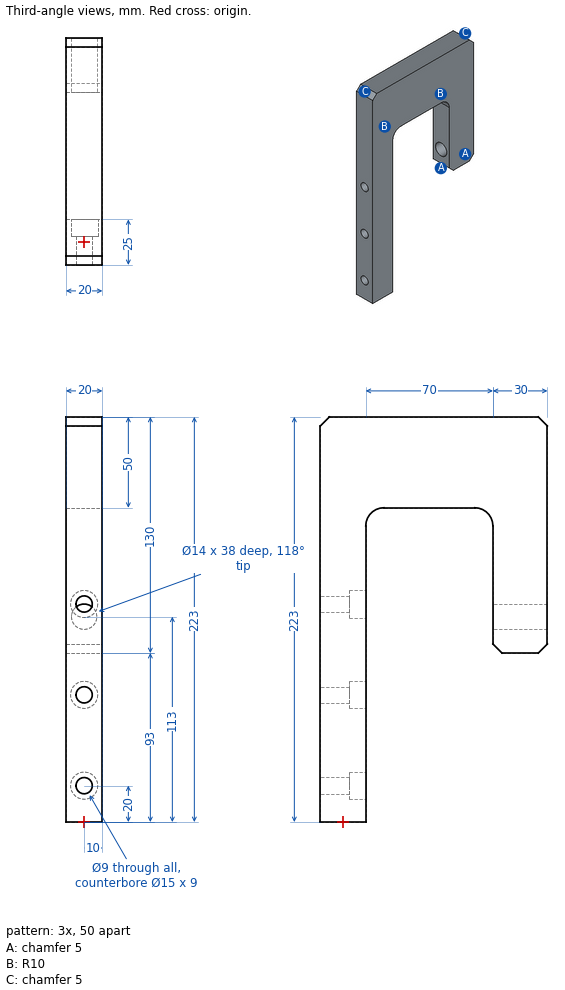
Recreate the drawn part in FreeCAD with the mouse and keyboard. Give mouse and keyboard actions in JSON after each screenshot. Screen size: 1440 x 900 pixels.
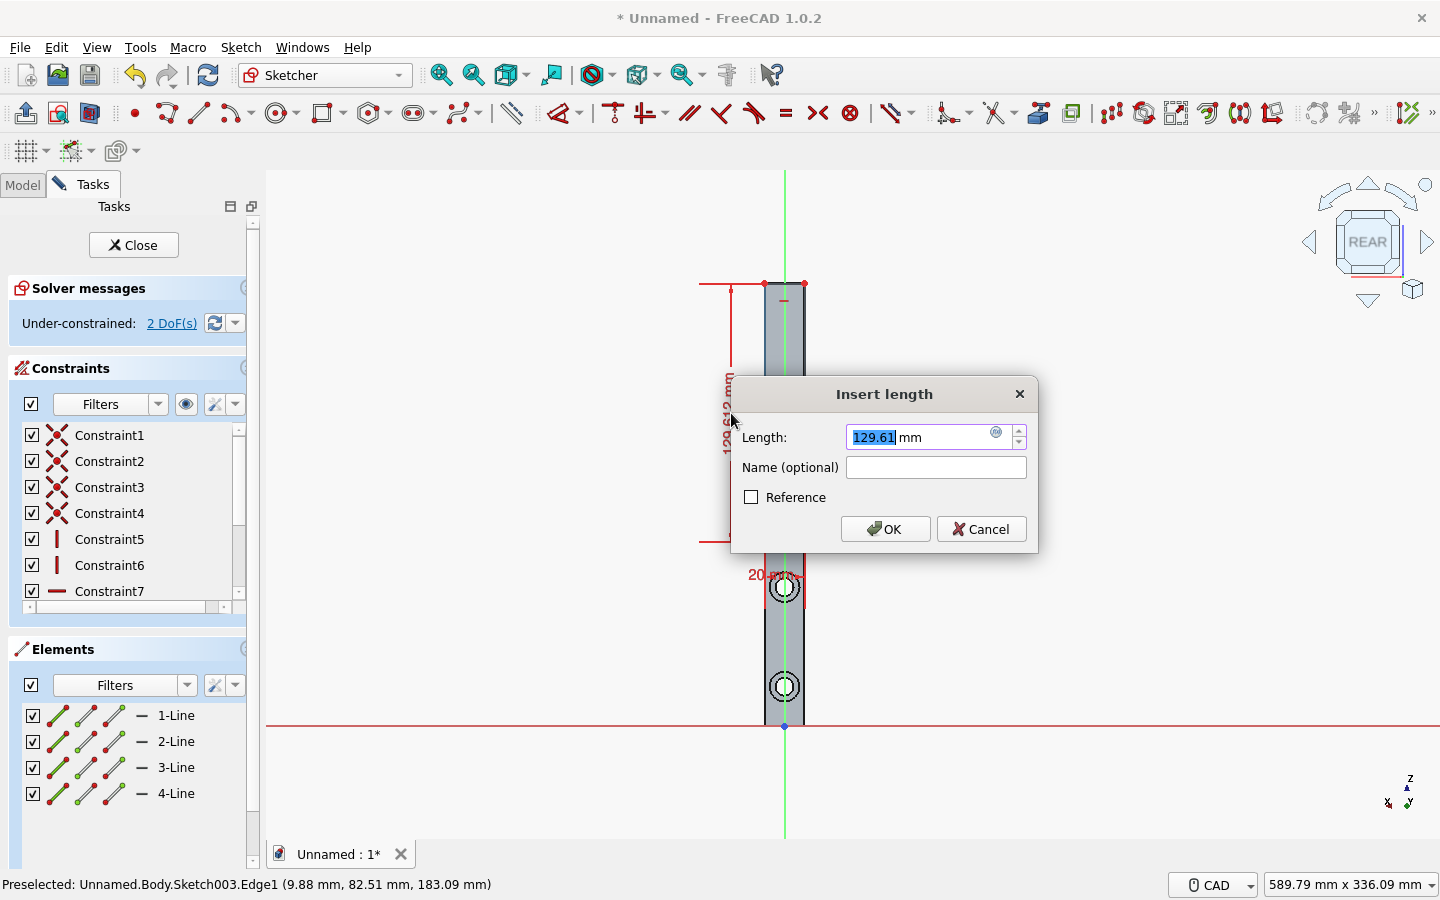
{"action": "type", "text": "130"}
{"action": "key", "text": "Return"}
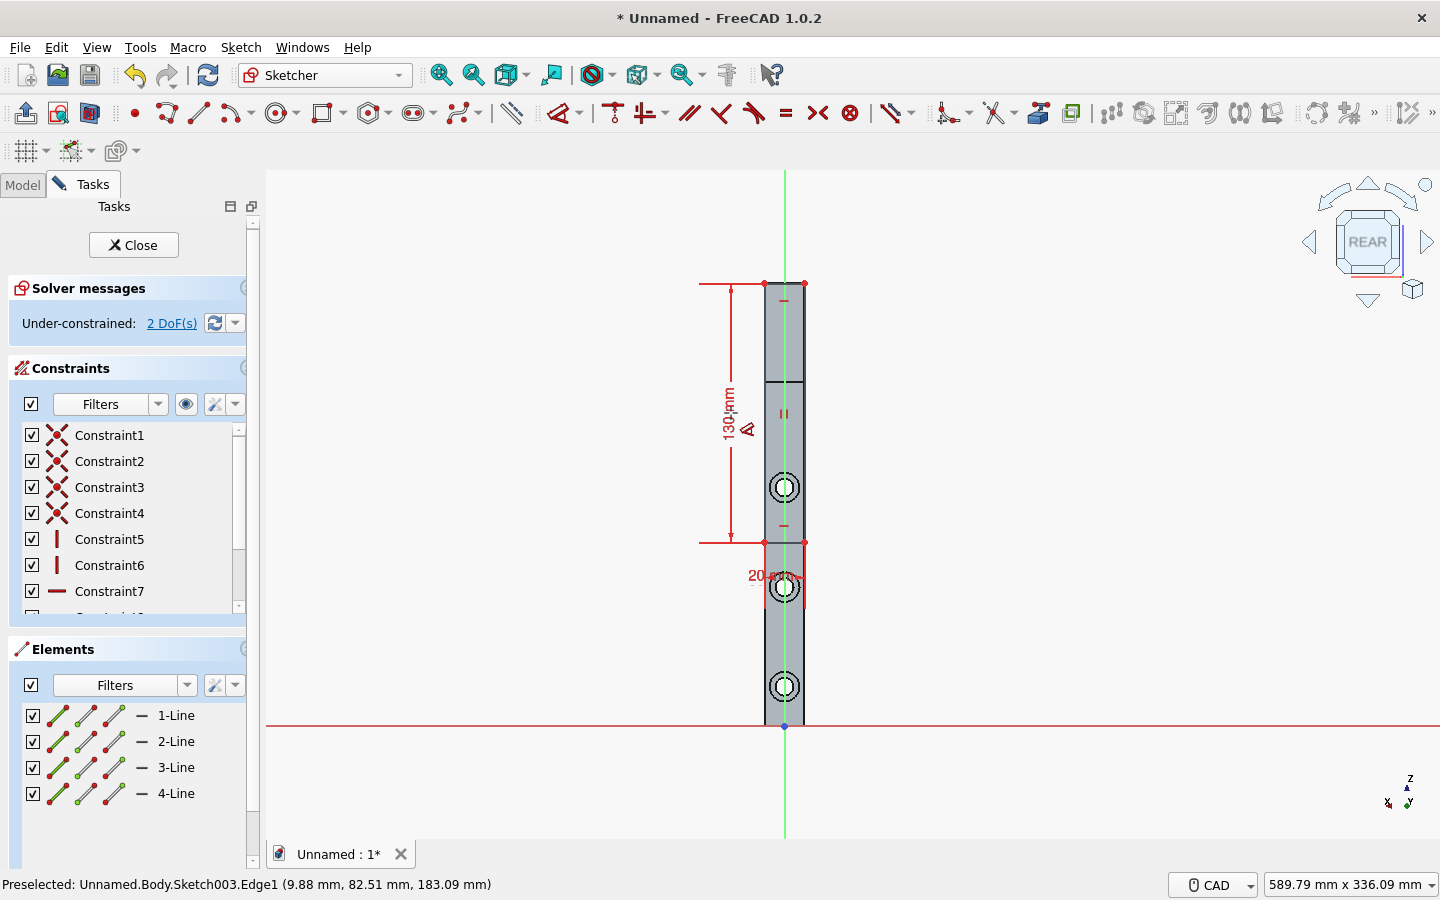
{"action": "scroll", "coordinate": [765, 284], "scroll_direction": "up", "scroll_amount": 4}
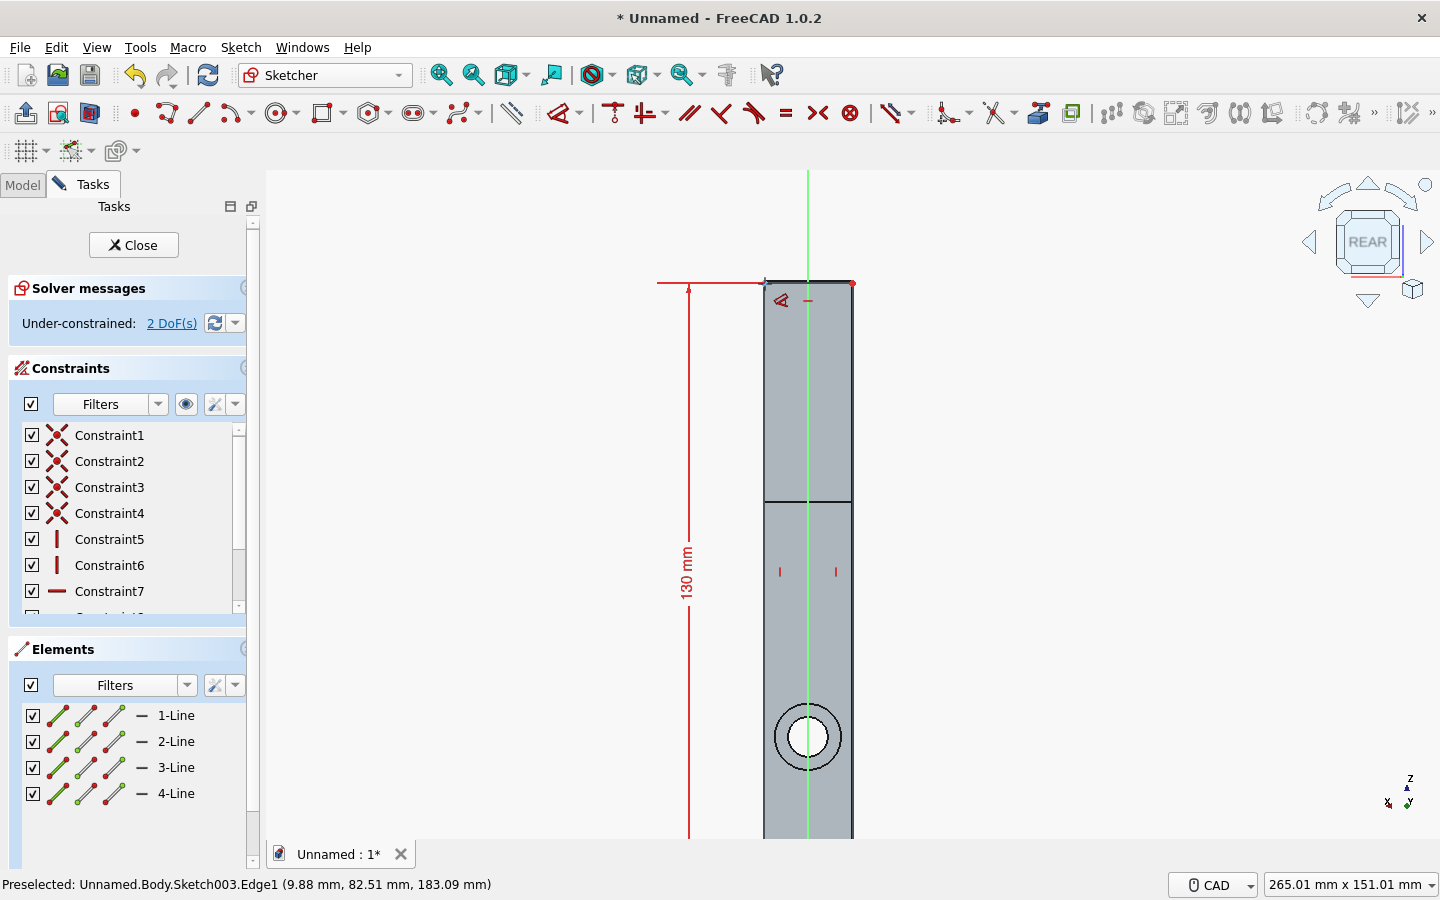
{"action": "left_click", "coordinate": [764, 283]}
{"action": "left_click", "coordinate": [786, 249]}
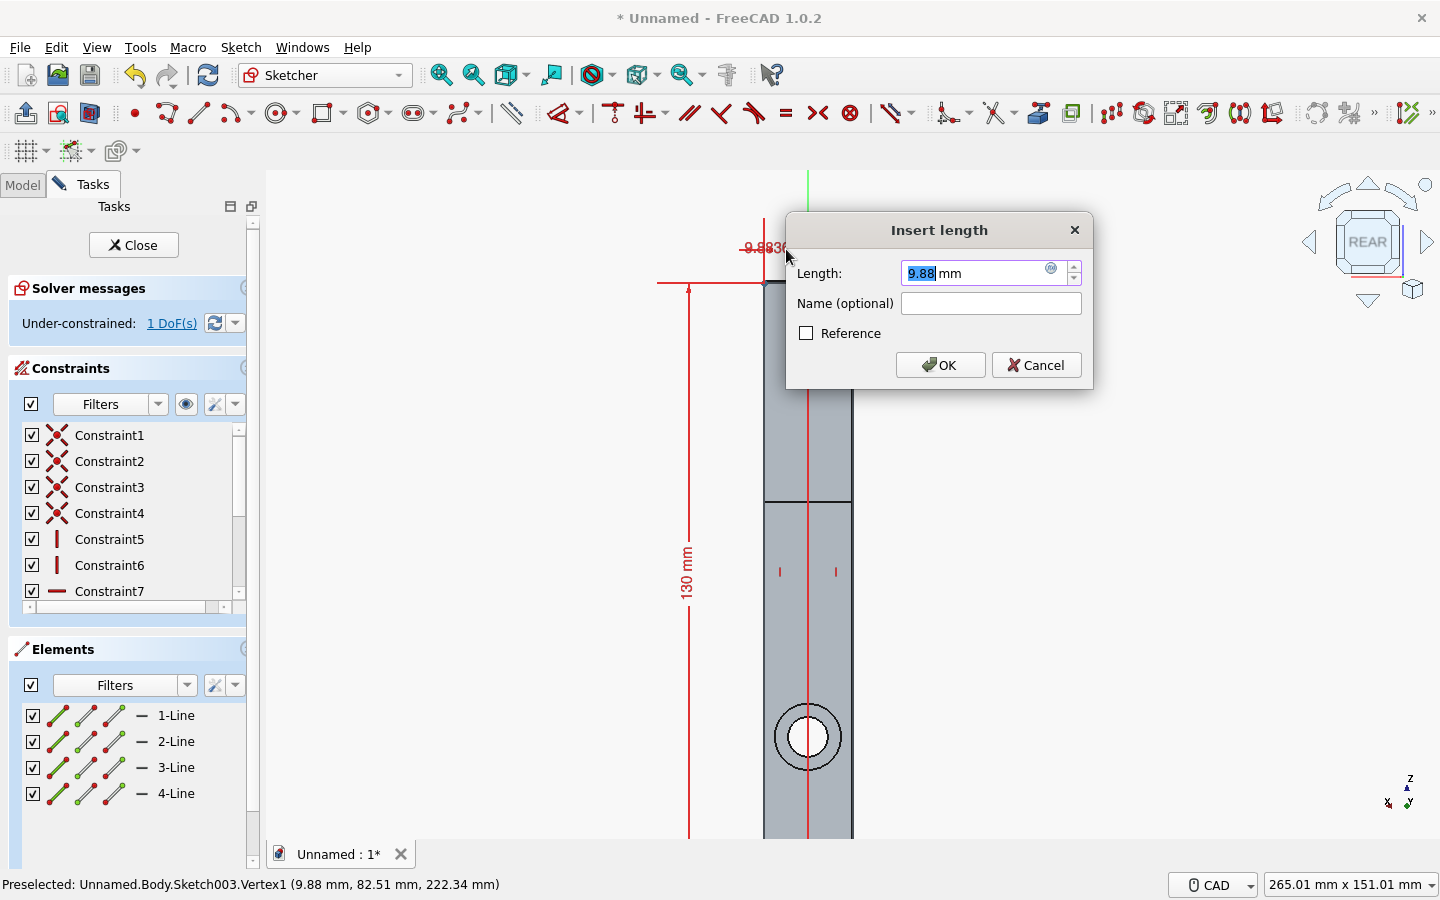
{"action": "type", "text": "10"}
{"action": "key", "text": "Return"}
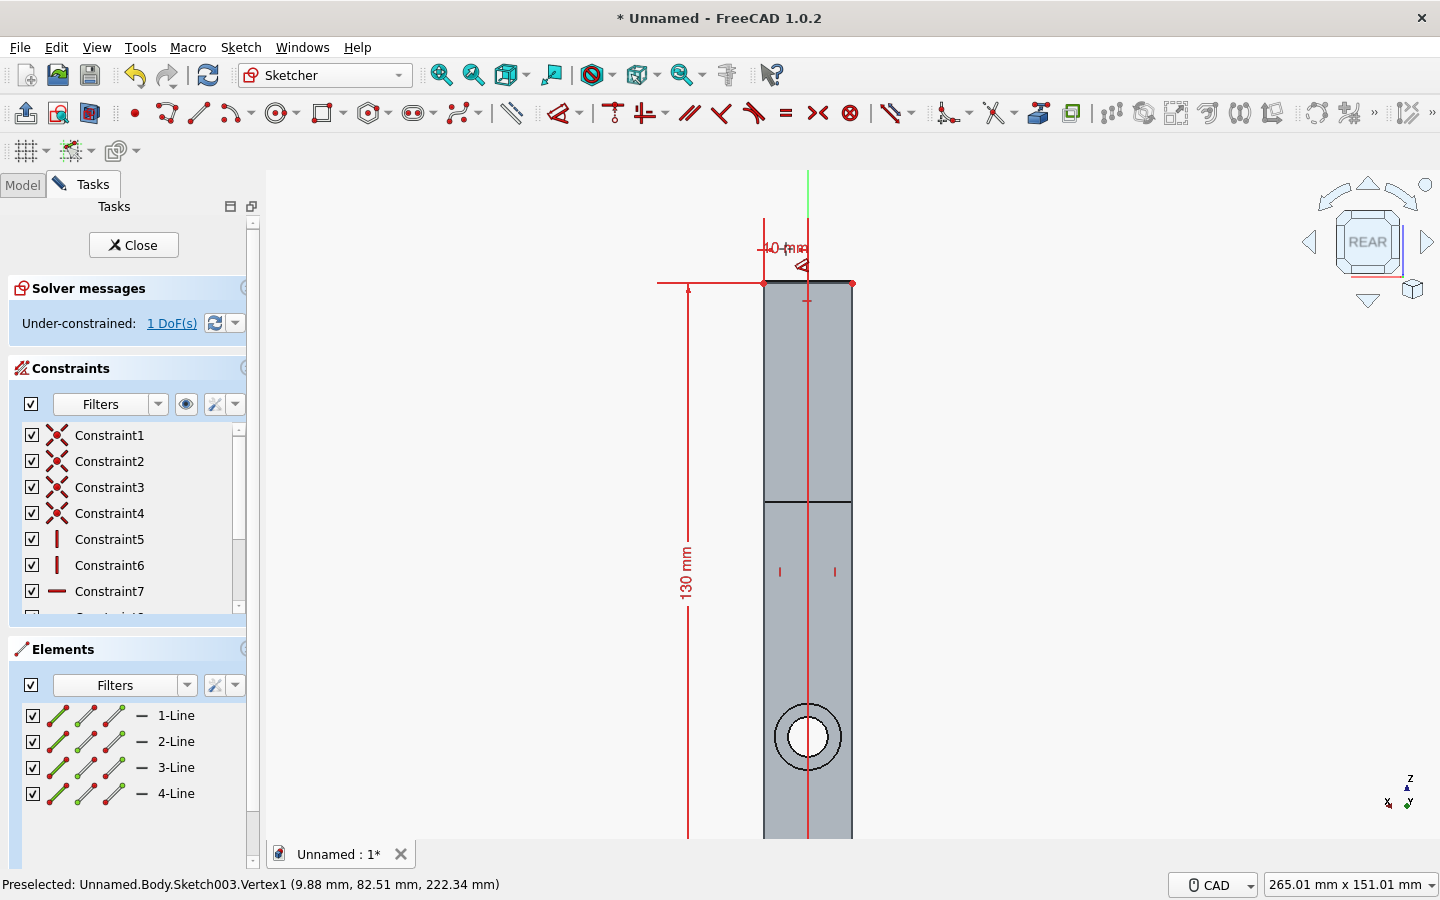
{"action": "scroll", "coordinate": [765, 284], "scroll_direction": "down", "scroll_amount": 4}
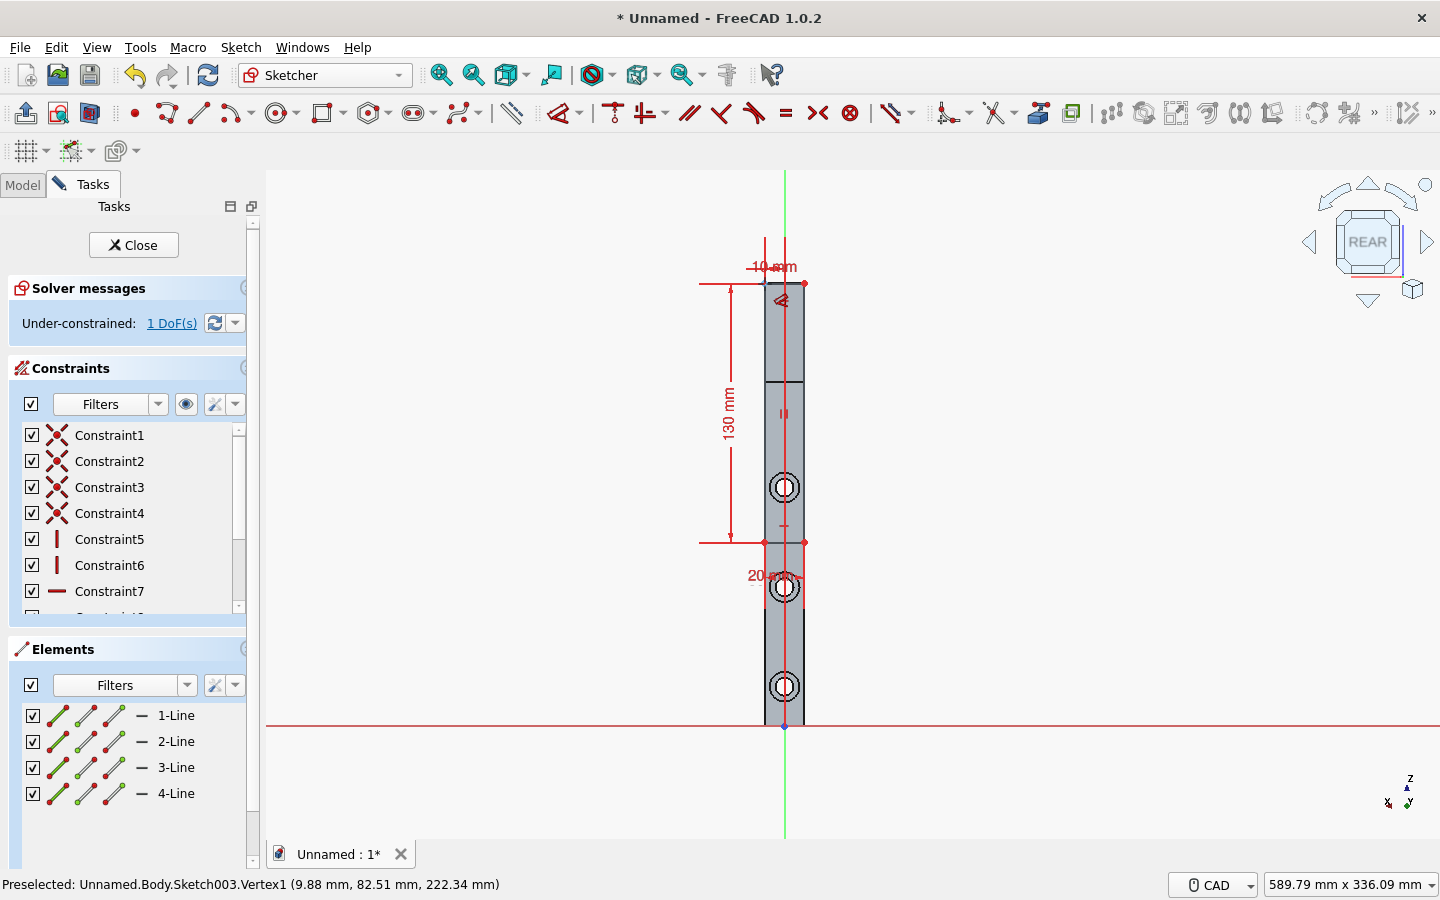
{"action": "left_click", "coordinate": [765, 543]}
{"action": "left_click", "coordinate": [731, 635]}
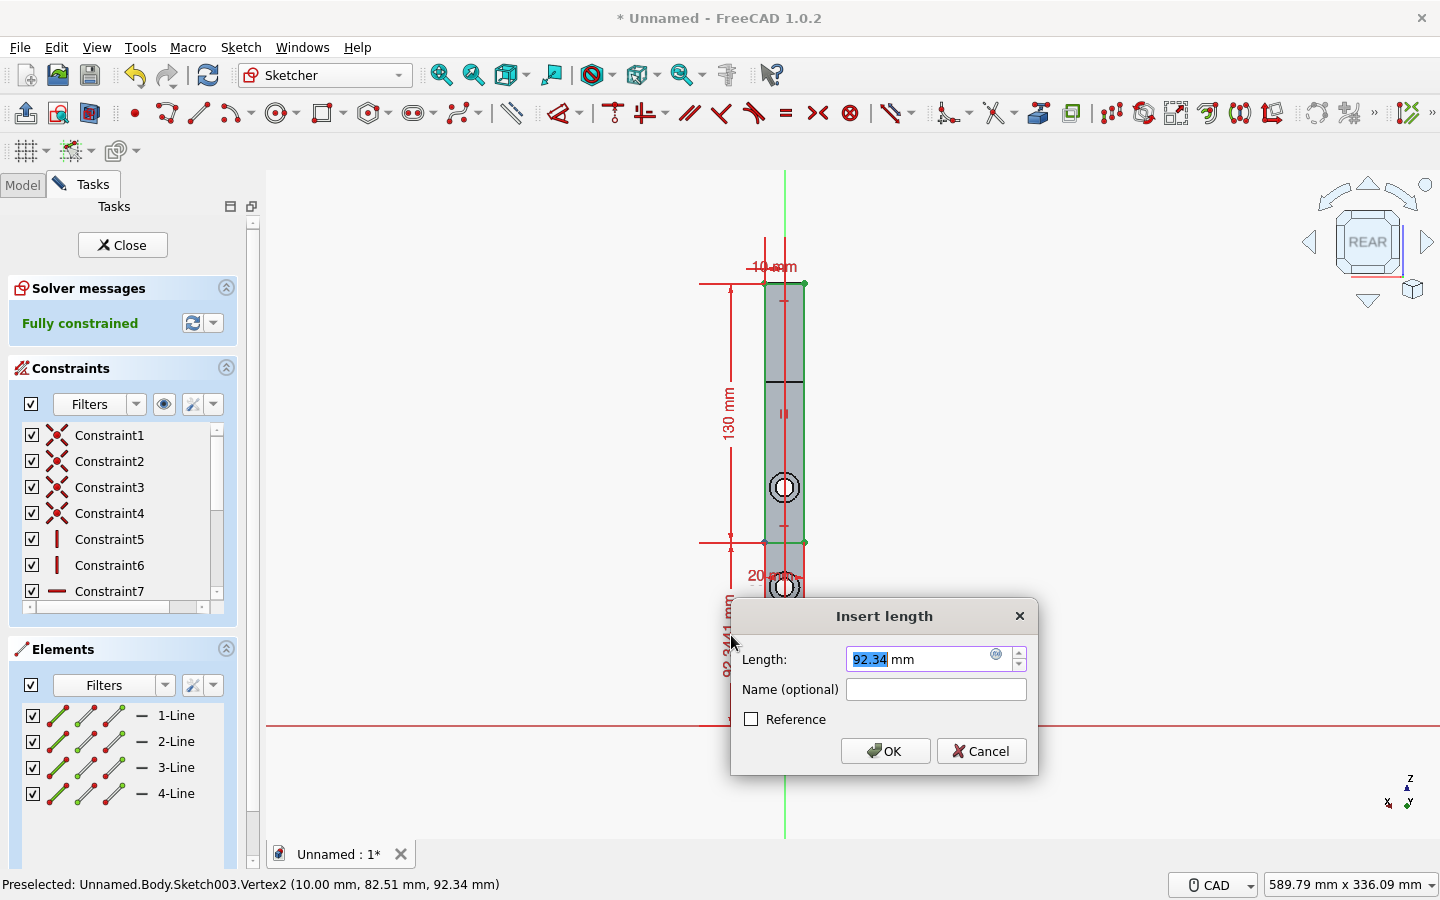
{"action": "type", "text": "93"}
{"action": "key", "text": "Return"}
{"action": "key", "text": "Escape"}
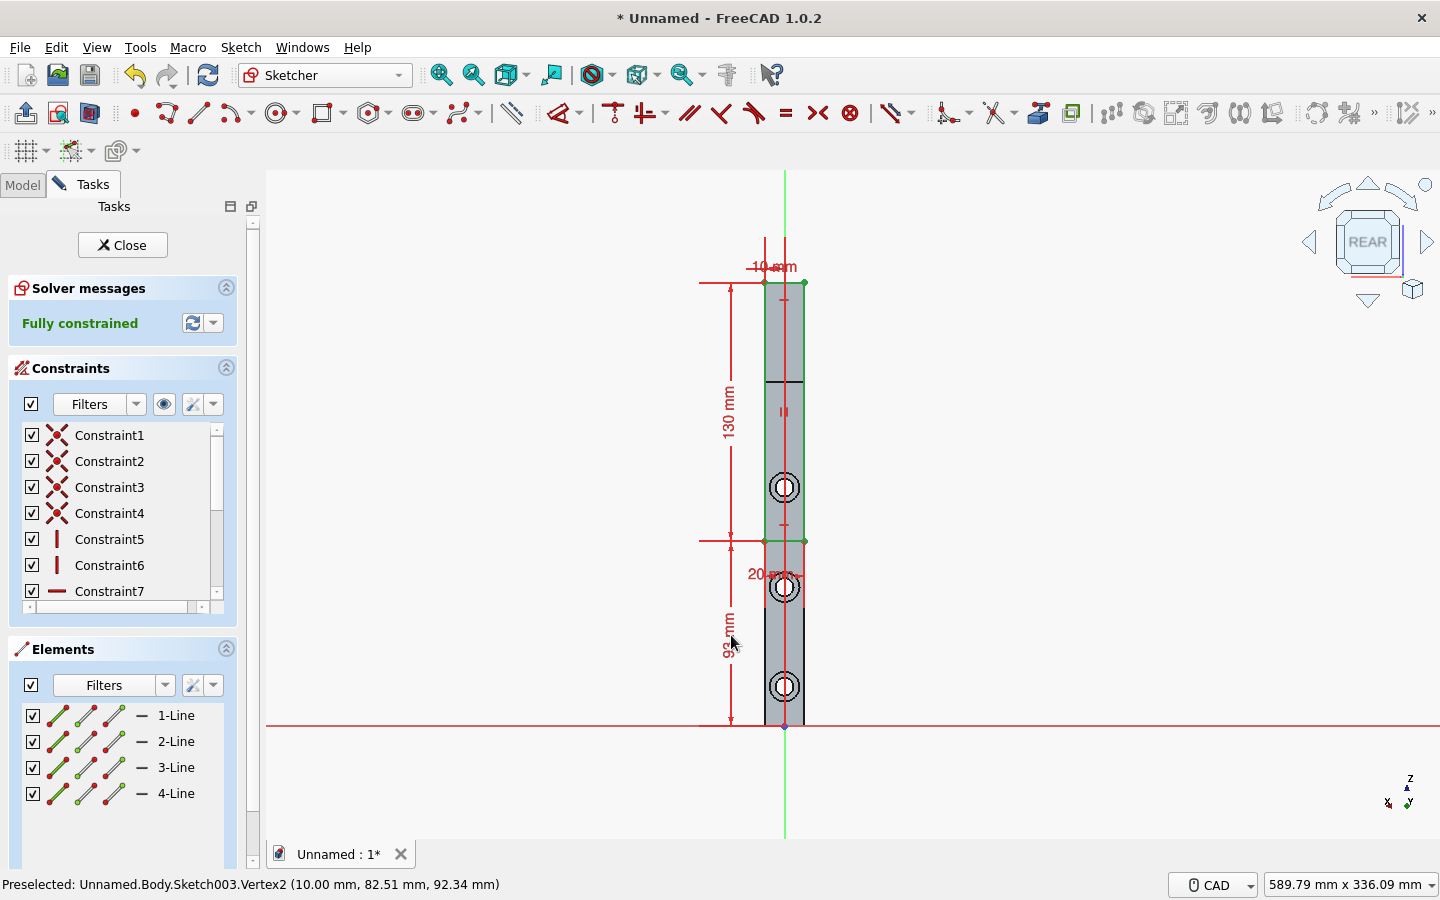
{"action": "left_click", "coordinate": [123, 245]}